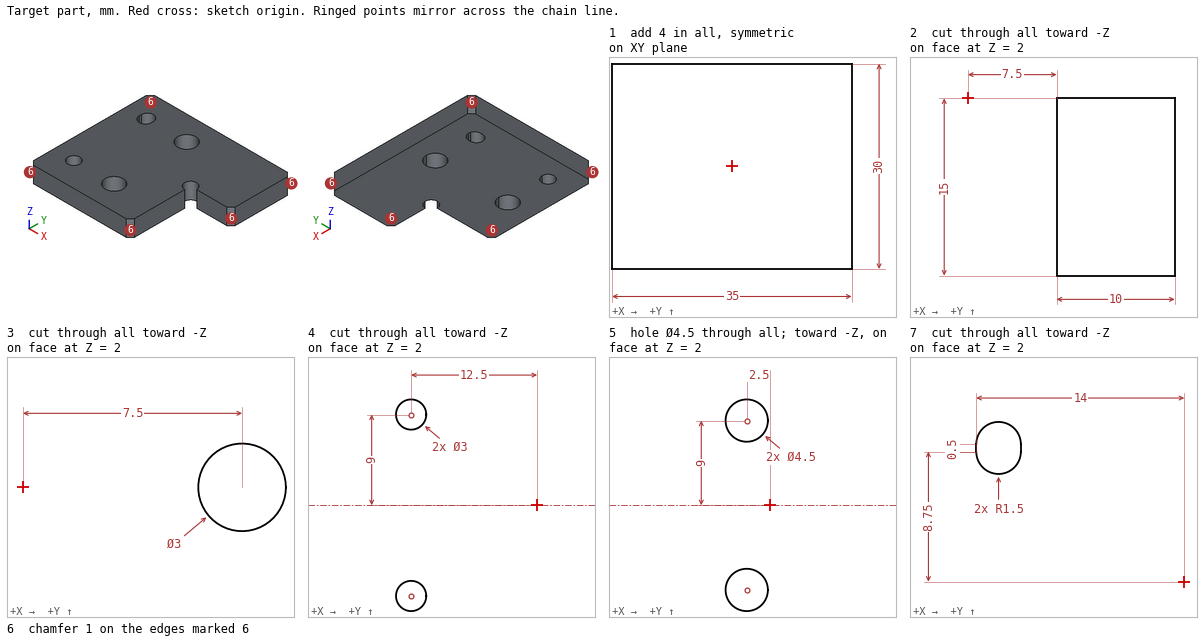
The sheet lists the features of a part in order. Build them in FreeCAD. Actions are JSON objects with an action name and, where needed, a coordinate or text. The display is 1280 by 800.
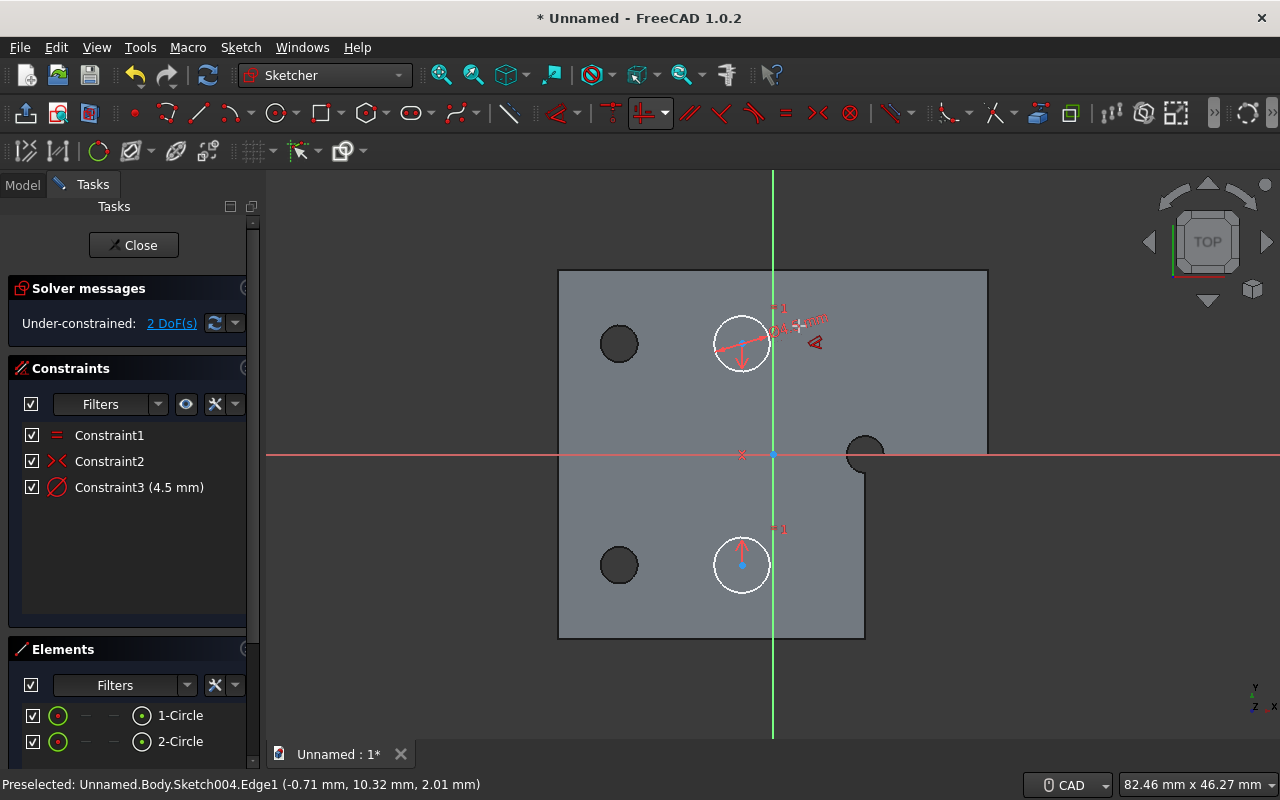
{"action": "left_click", "coordinate": [742, 344]}
{"action": "left_click", "coordinate": [807, 399]}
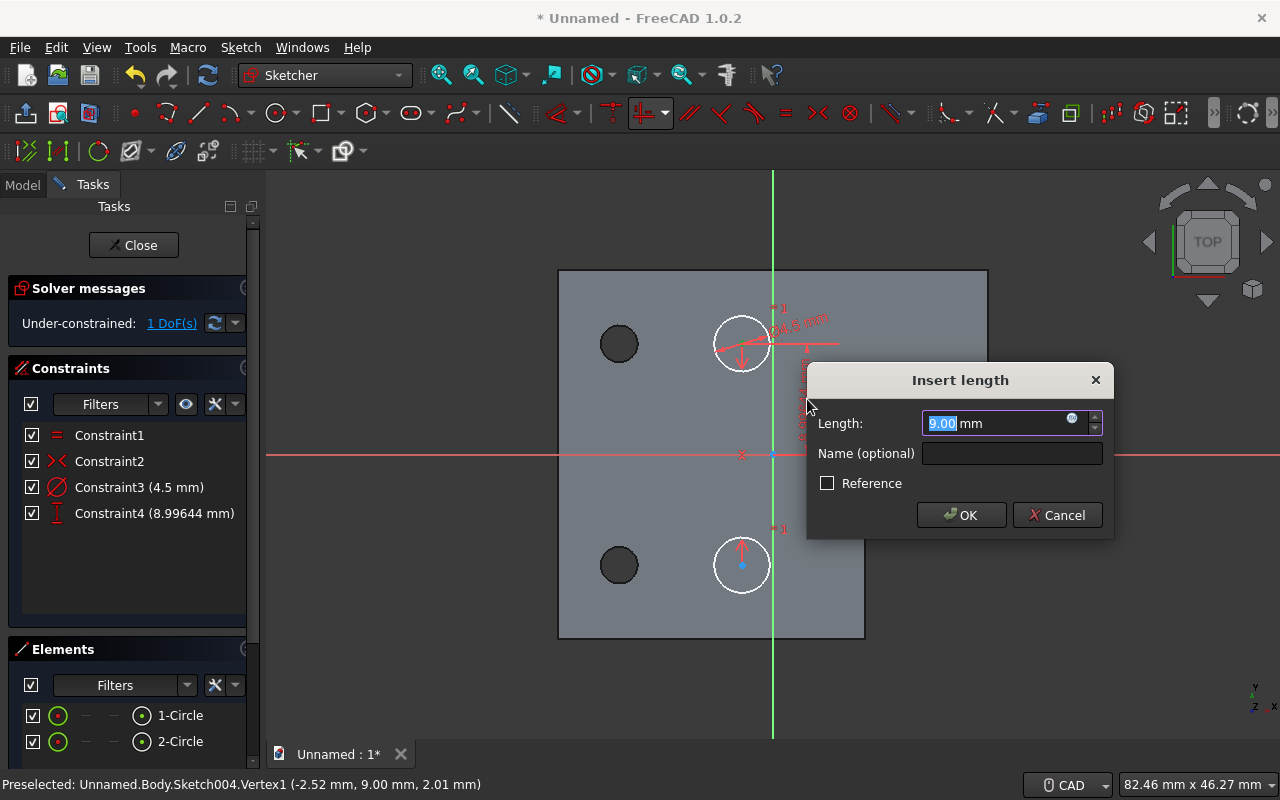
{"action": "type", "text": "9"}
{"action": "key", "text": "Return"}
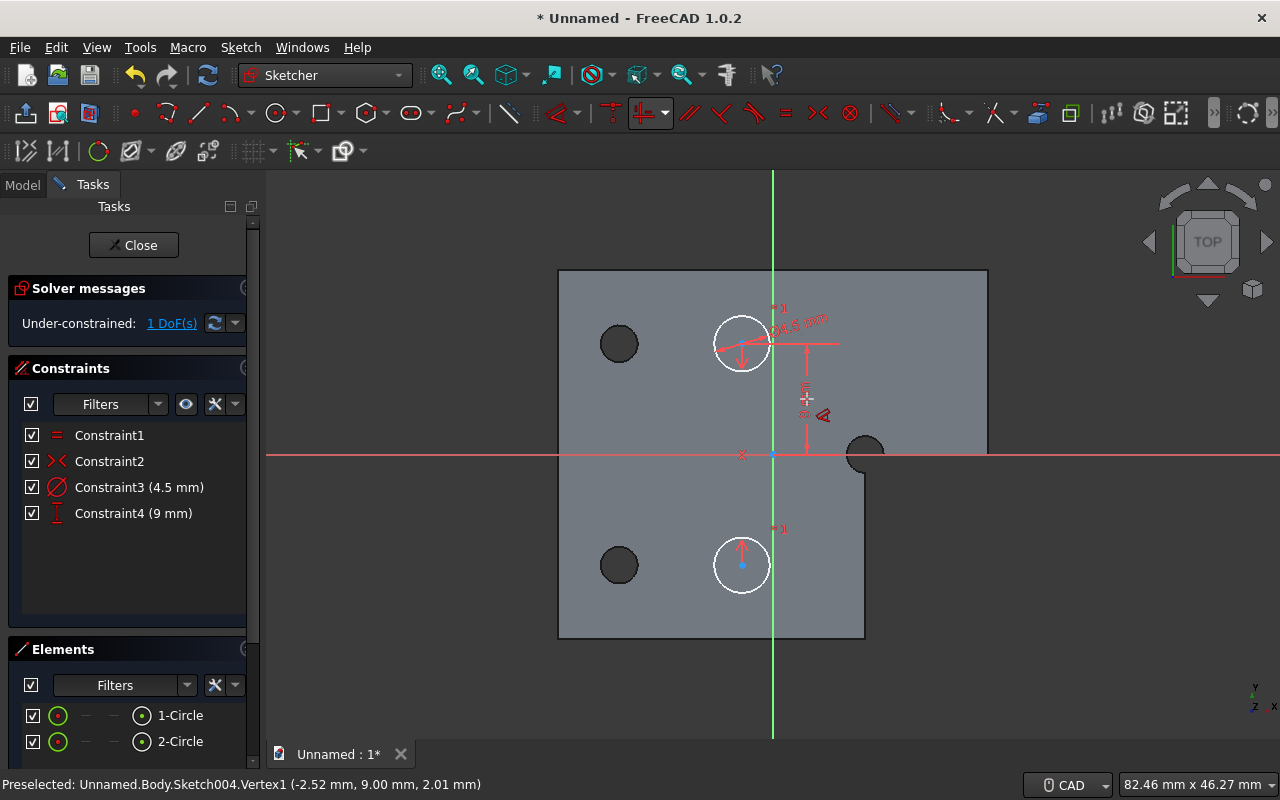
{"action": "scroll", "coordinate": [742, 344], "scroll_direction": "up", "scroll_amount": 2}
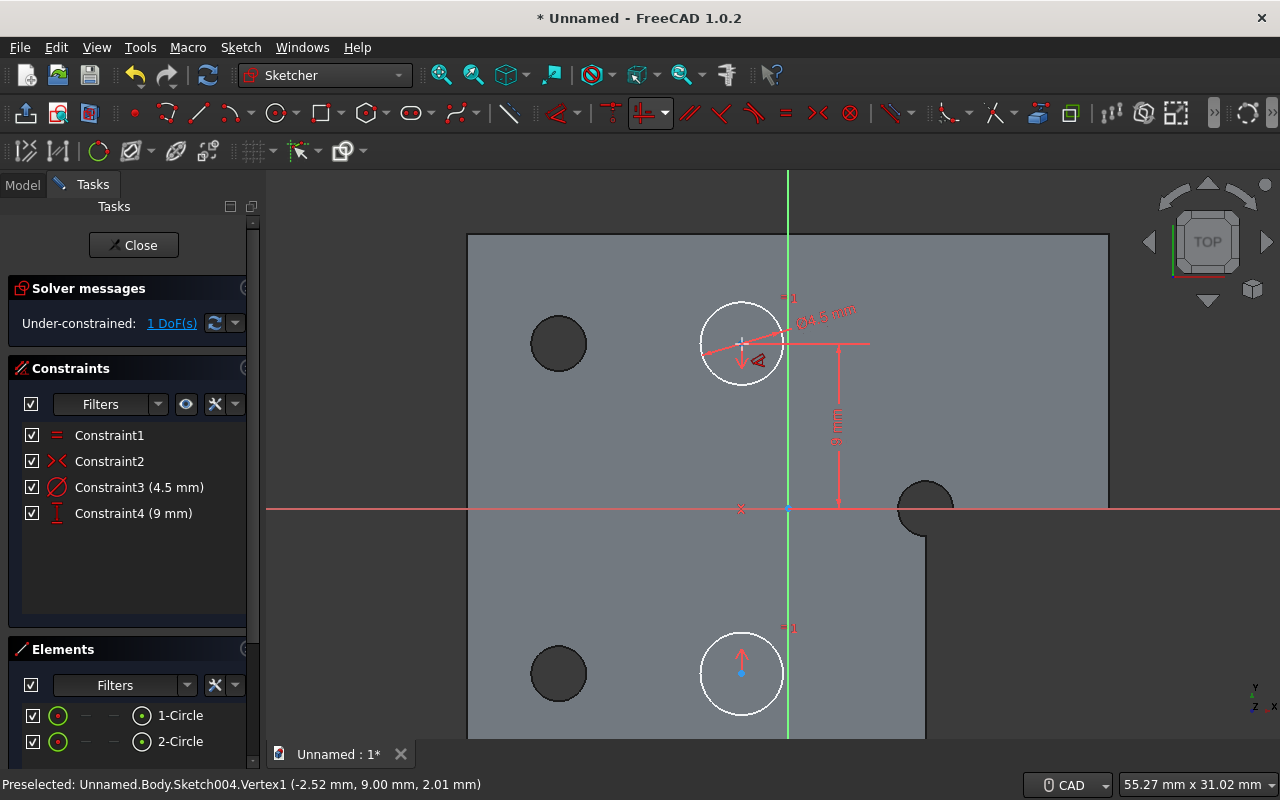
{"action": "left_click", "coordinate": [742, 344]}
{"action": "left_click", "coordinate": [765, 543]}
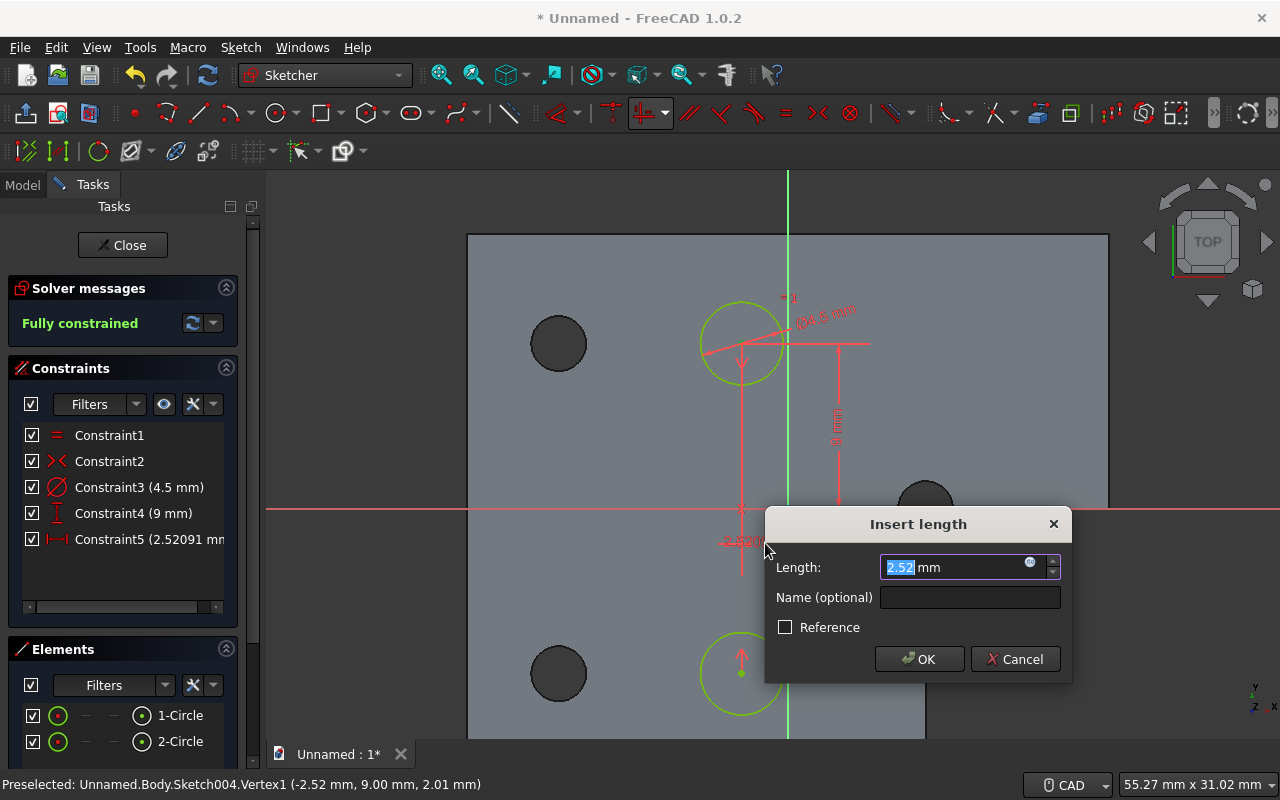
{"action": "type", "text": "2.5"}
{"action": "key", "text": "Return"}
{"action": "key", "text": "Escape"}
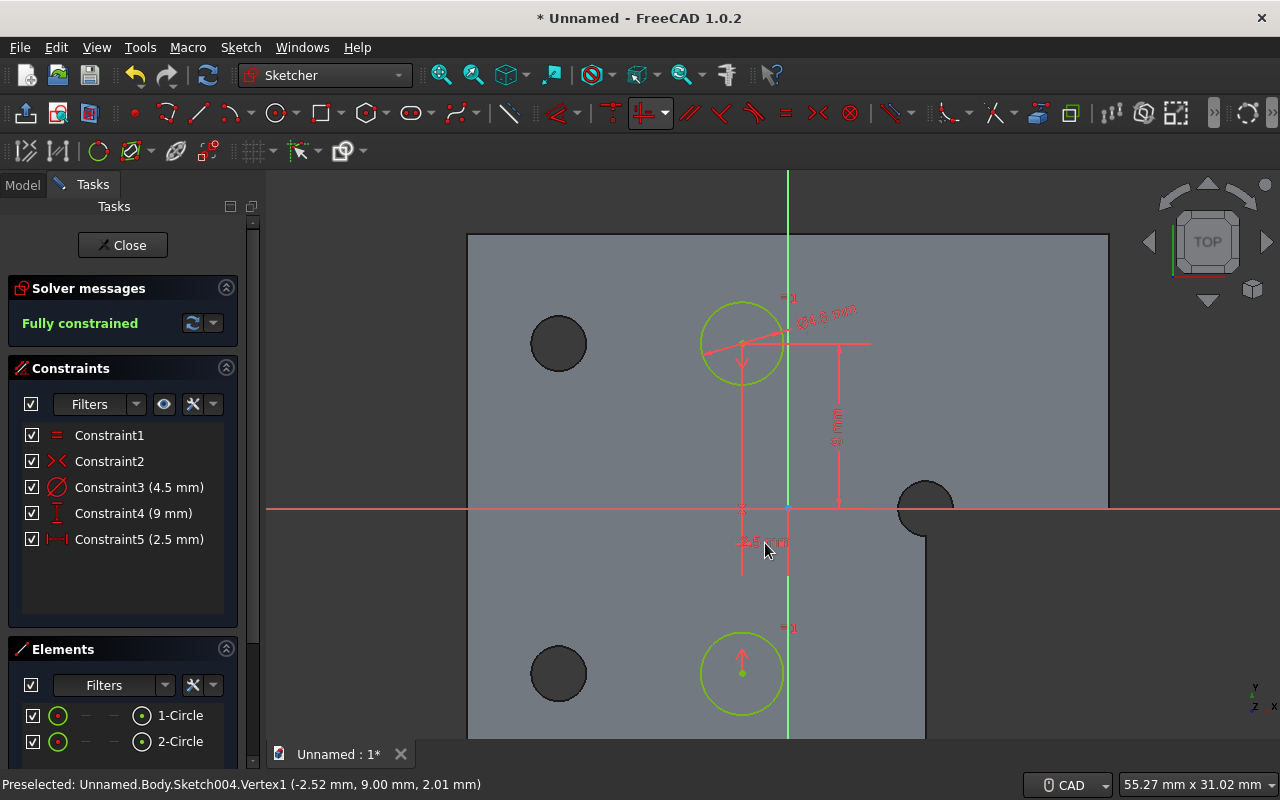
{"action": "left_click", "coordinate": [123, 245]}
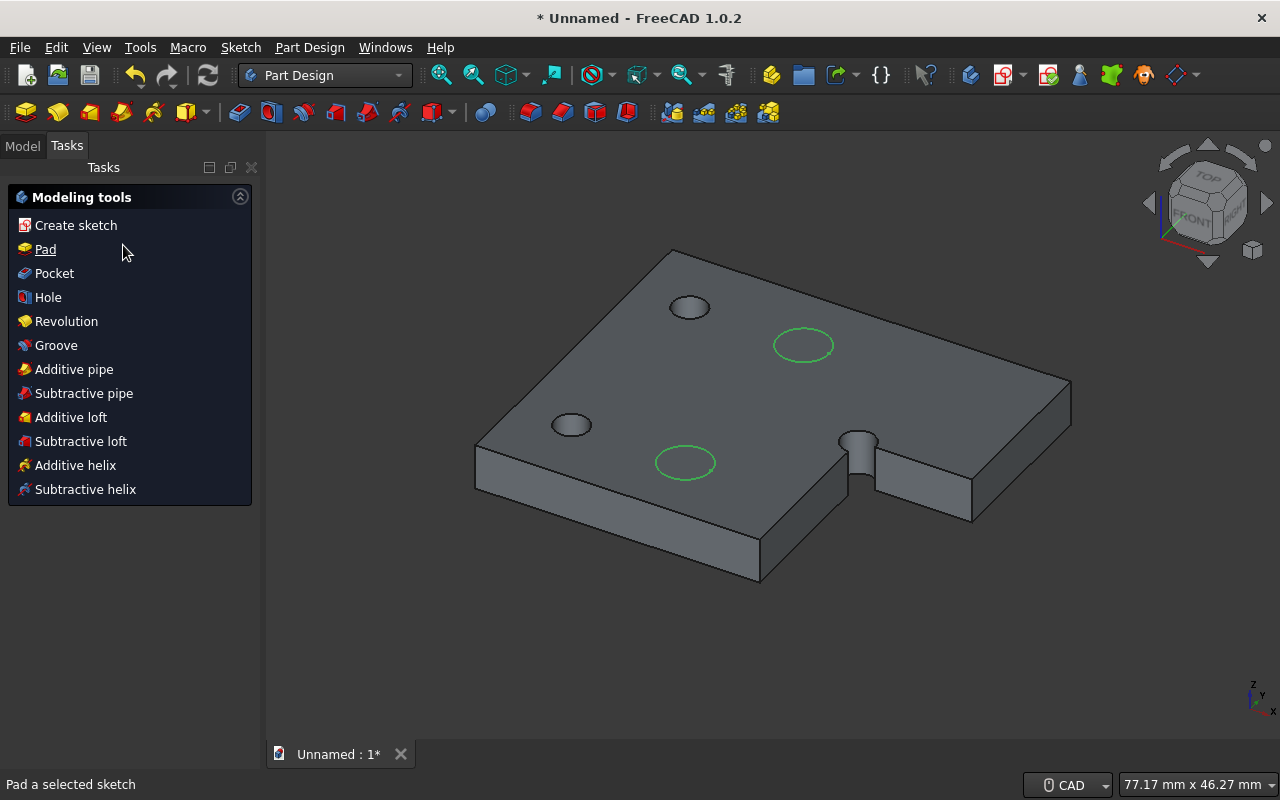
{"action": "left_click", "coordinate": [272, 112]}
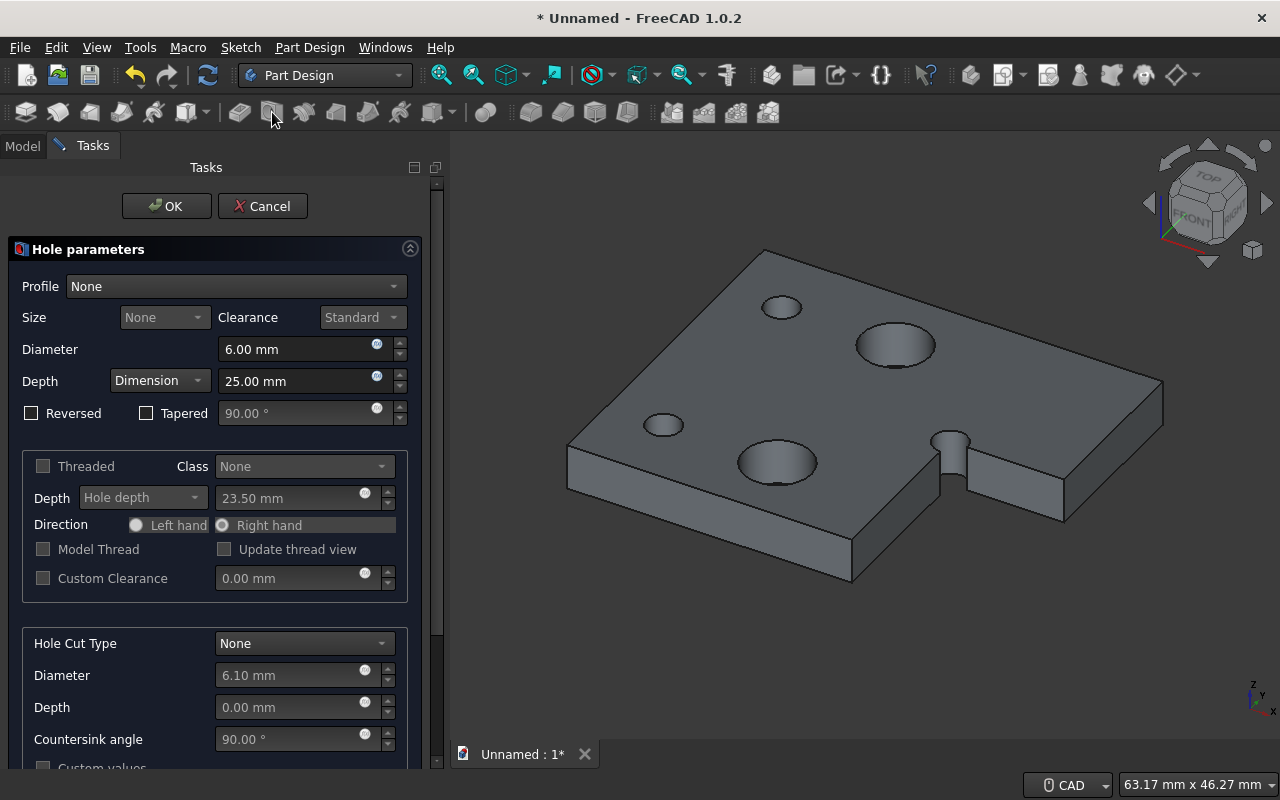
{"action": "triple_click", "coordinate": [305, 349]}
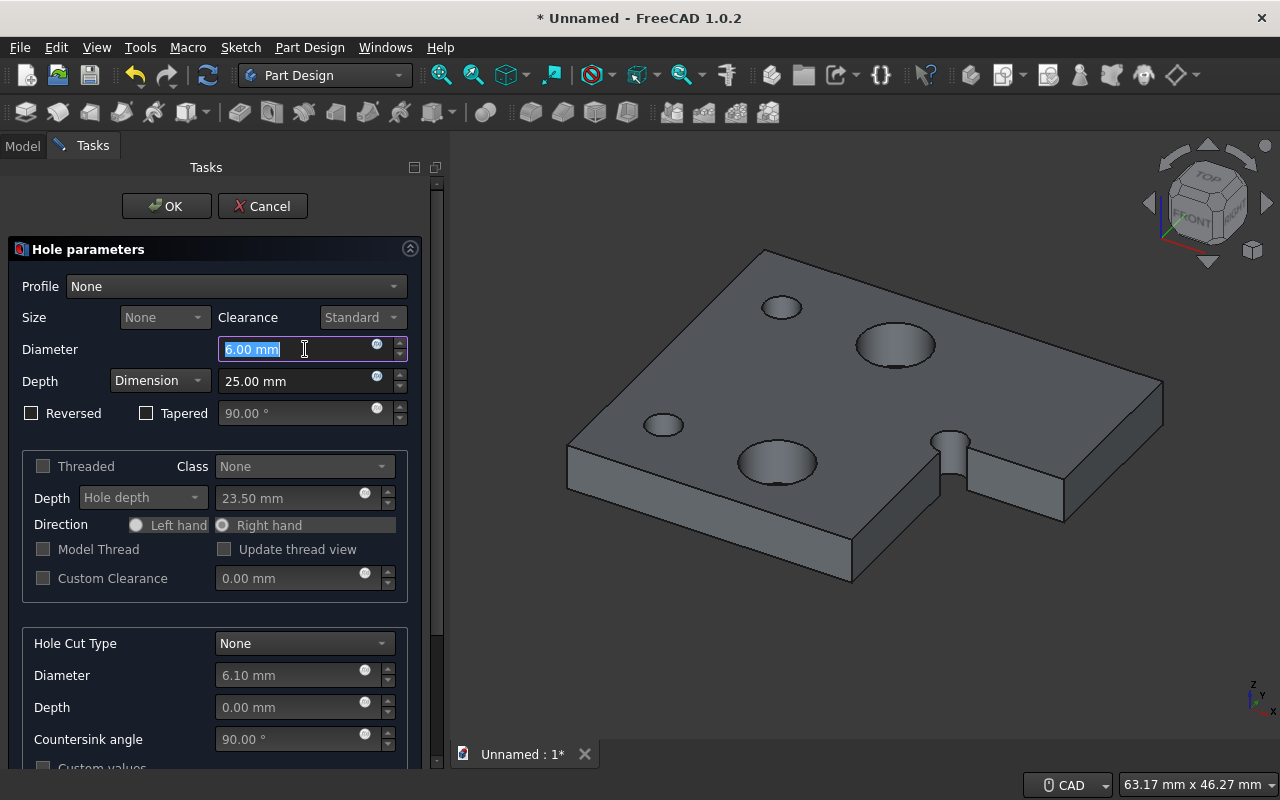
{"action": "type", "text": "4.5"}
{"action": "key", "text": "Tab"}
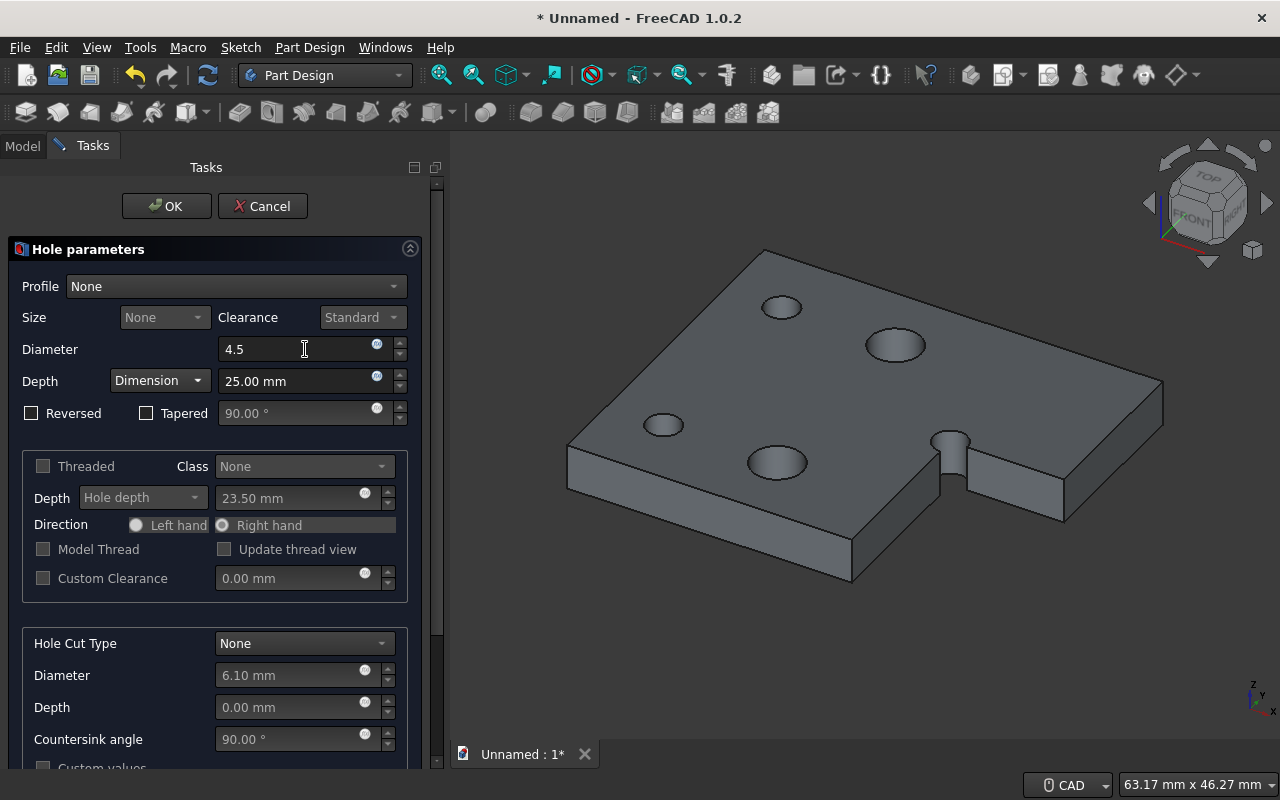
{"action": "left_click", "coordinate": [161, 380]}